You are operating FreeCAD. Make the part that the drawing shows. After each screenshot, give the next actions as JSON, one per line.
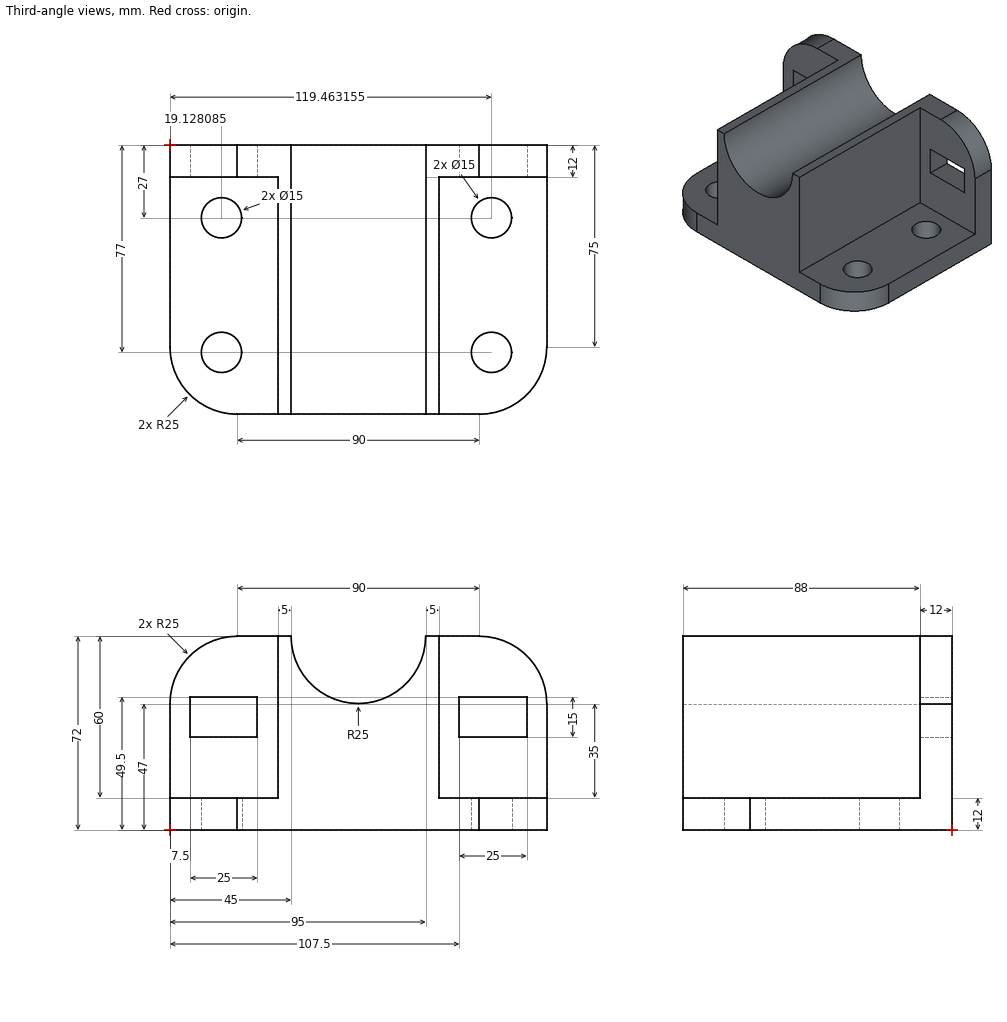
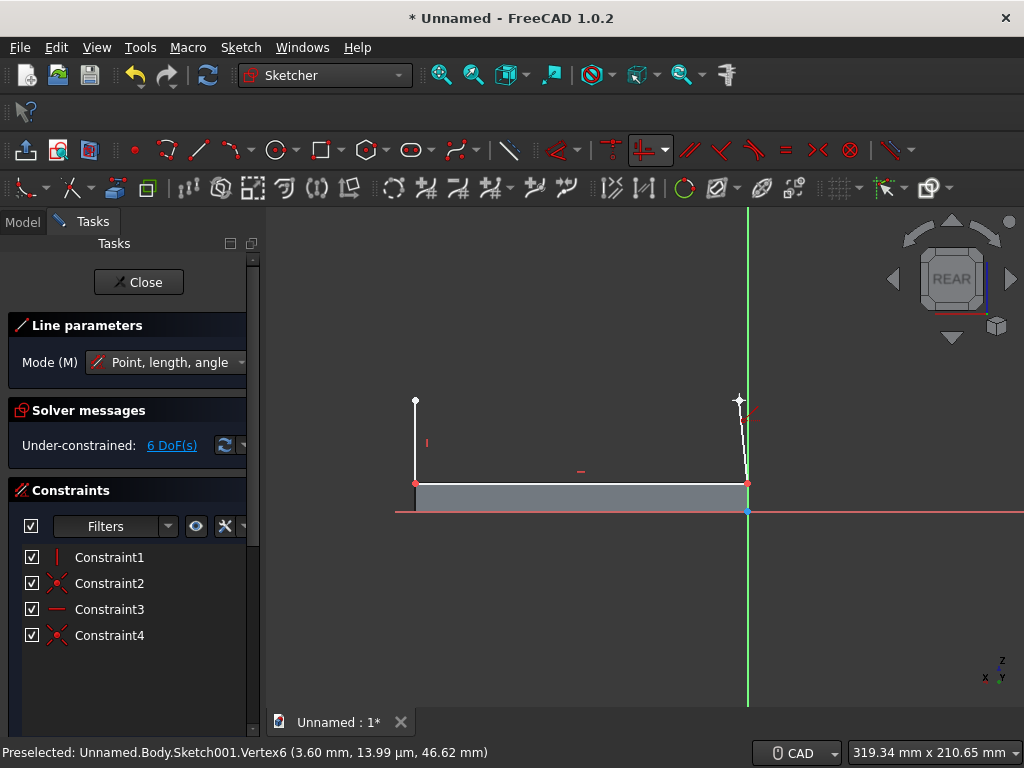
{"action": "left_click", "coordinate": [688, 341]}
{"action": "left_click", "coordinate": [475, 341]}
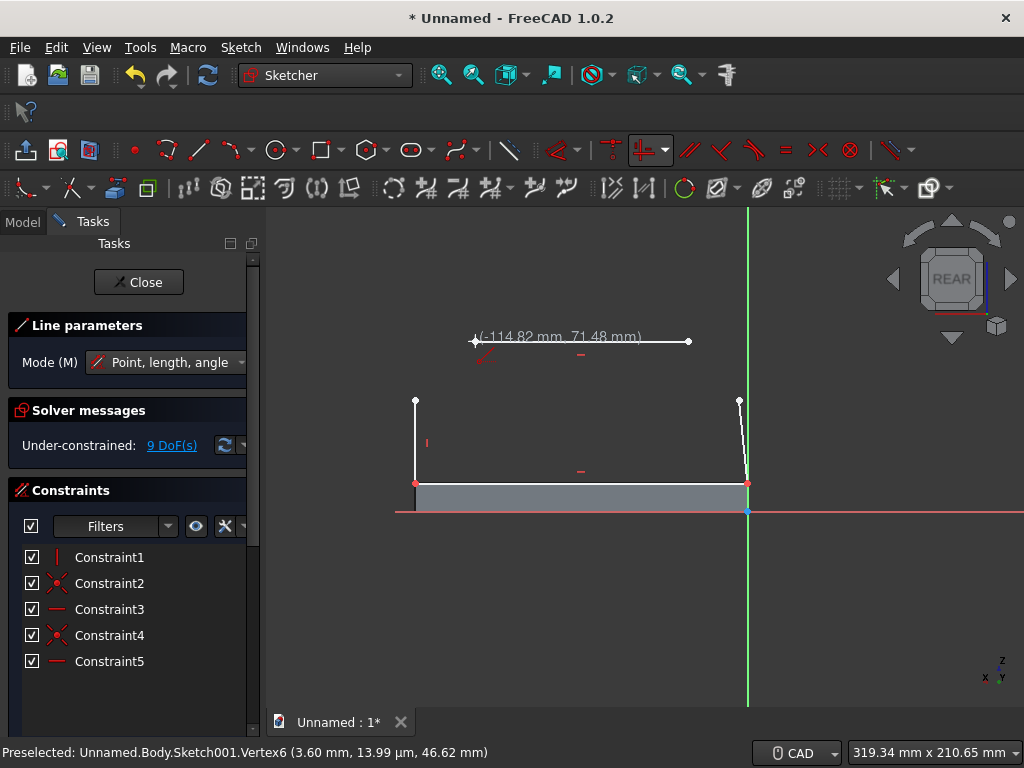
{"action": "left_click", "coordinate": [232, 150]}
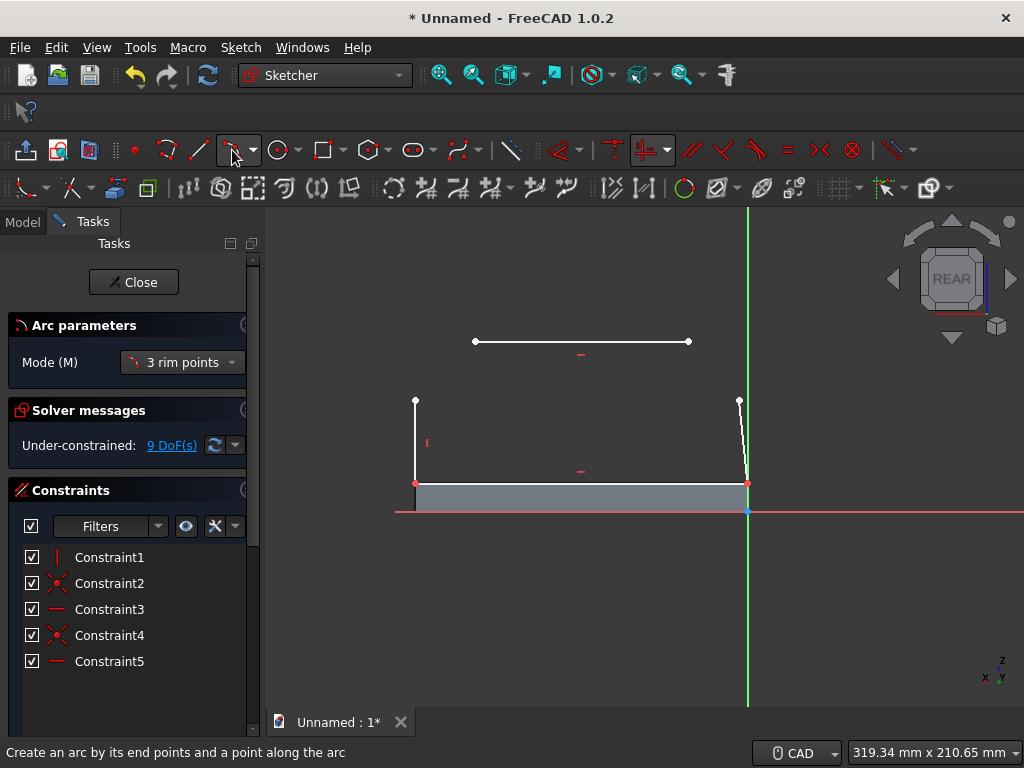
{"action": "left_click", "coordinate": [739, 401]}
{"action": "left_click", "coordinate": [688, 342]}
{"action": "left_click", "coordinate": [730, 358]}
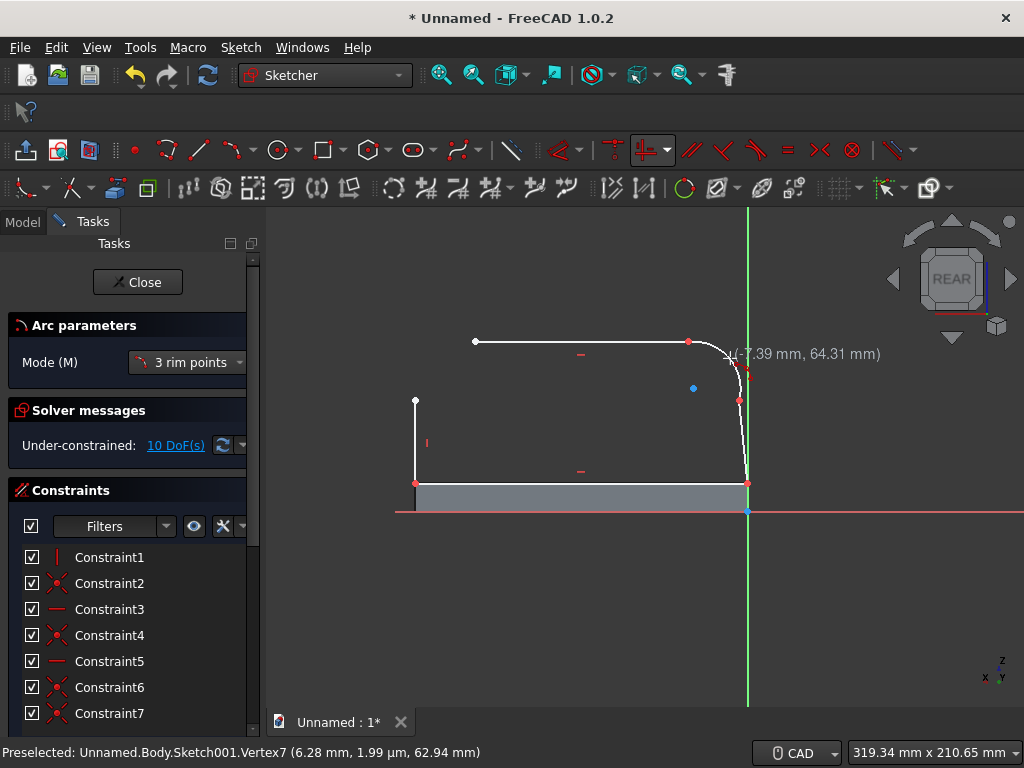
{"action": "left_click", "coordinate": [475, 342]}
{"action": "left_click", "coordinate": [415, 401]}
{"action": "left_click", "coordinate": [433, 358]}
{"action": "key", "text": "Escape"}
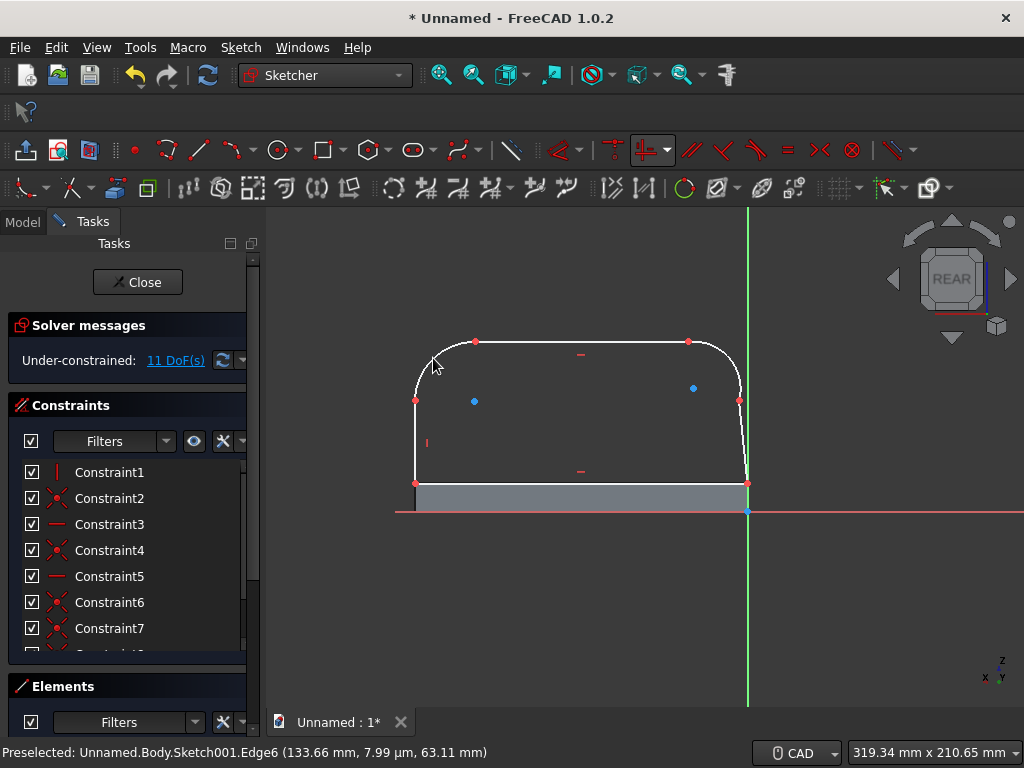
{"action": "left_click", "coordinate": [415, 426]}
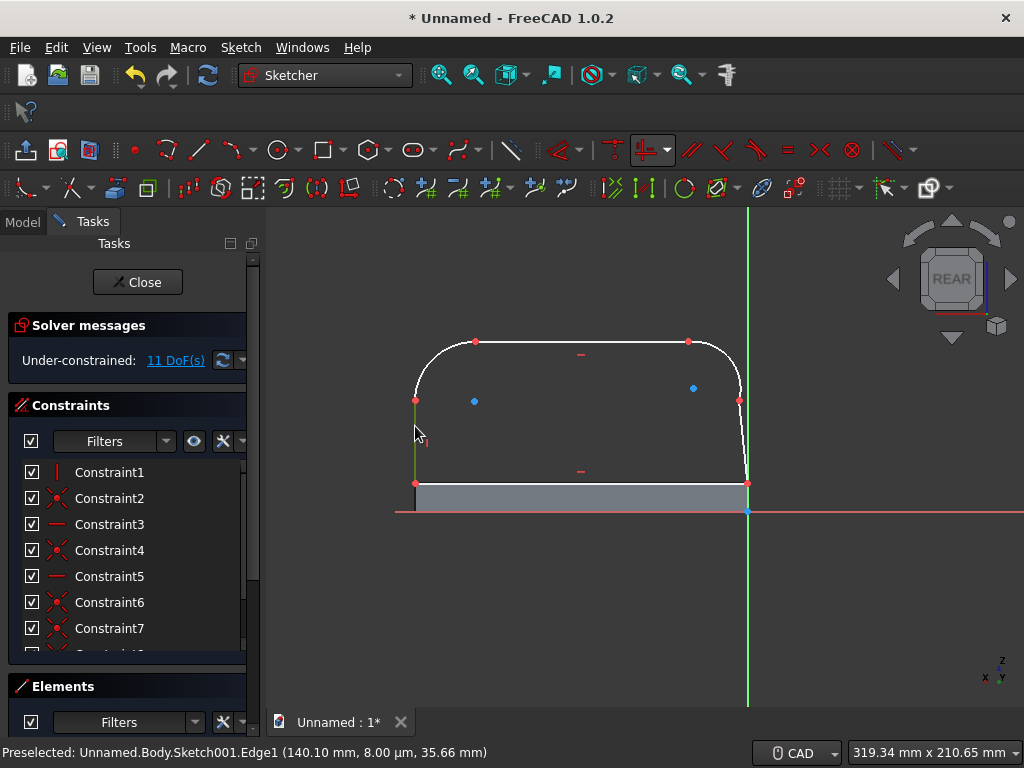
{"action": "left_click", "coordinate": [448, 348]}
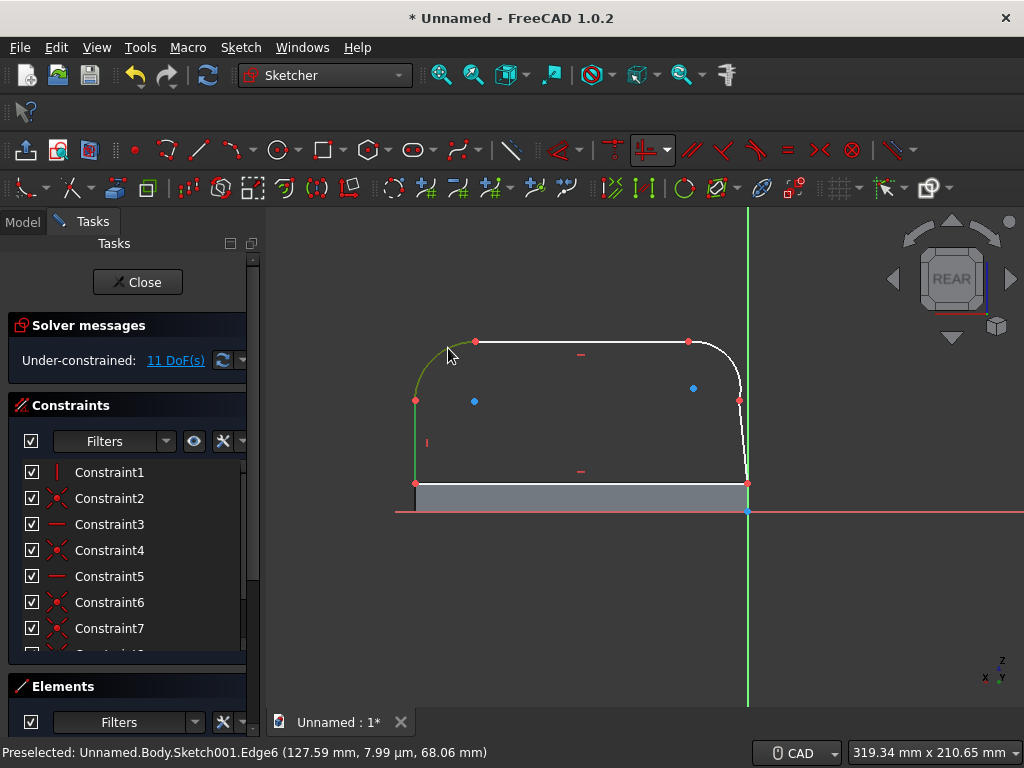
{"action": "key", "text": "t"}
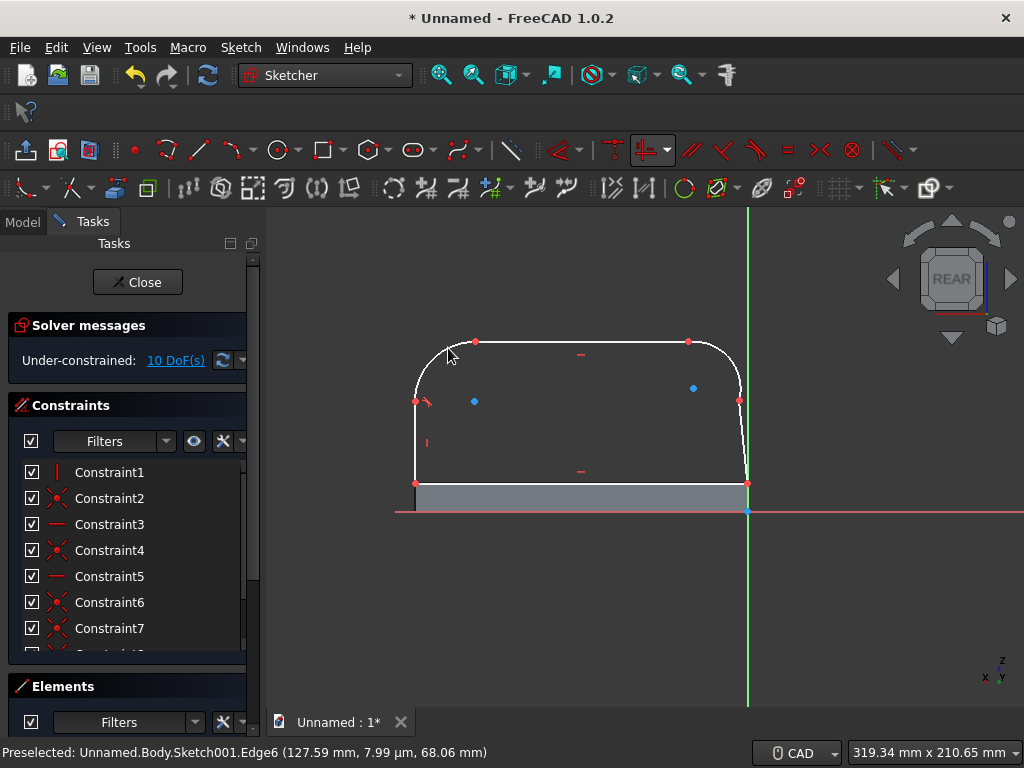
{"action": "left_click", "coordinate": [745, 459]}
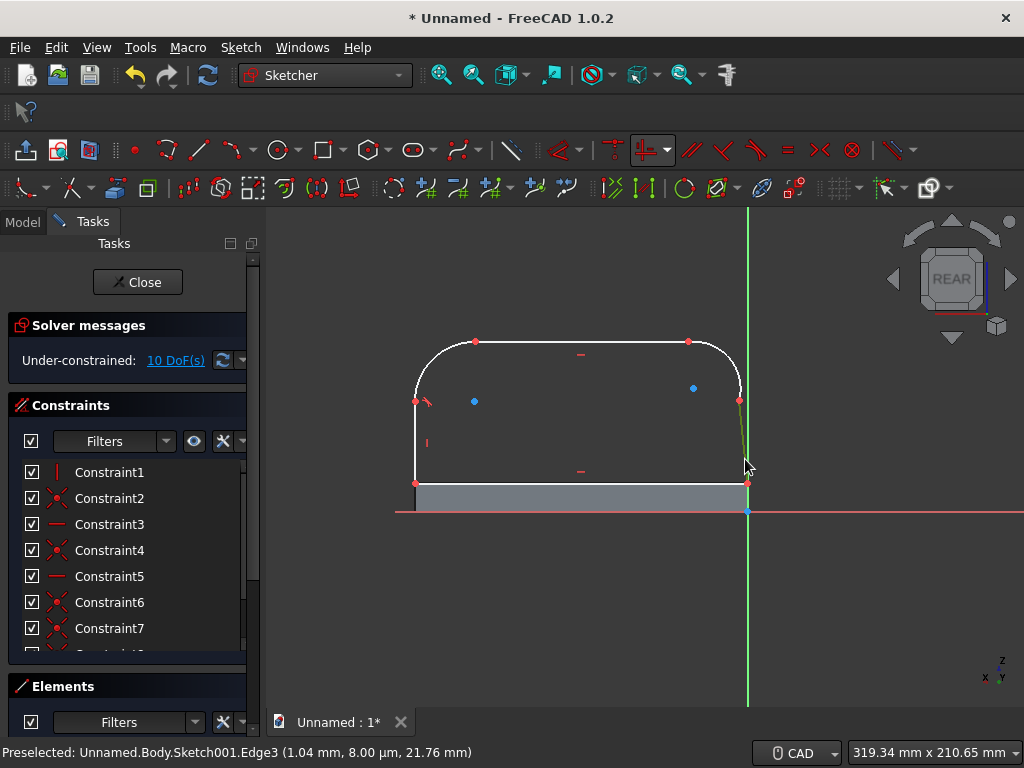
{"action": "scroll", "coordinate": [738, 374], "scroll_direction": "up", "scroll_amount": 2}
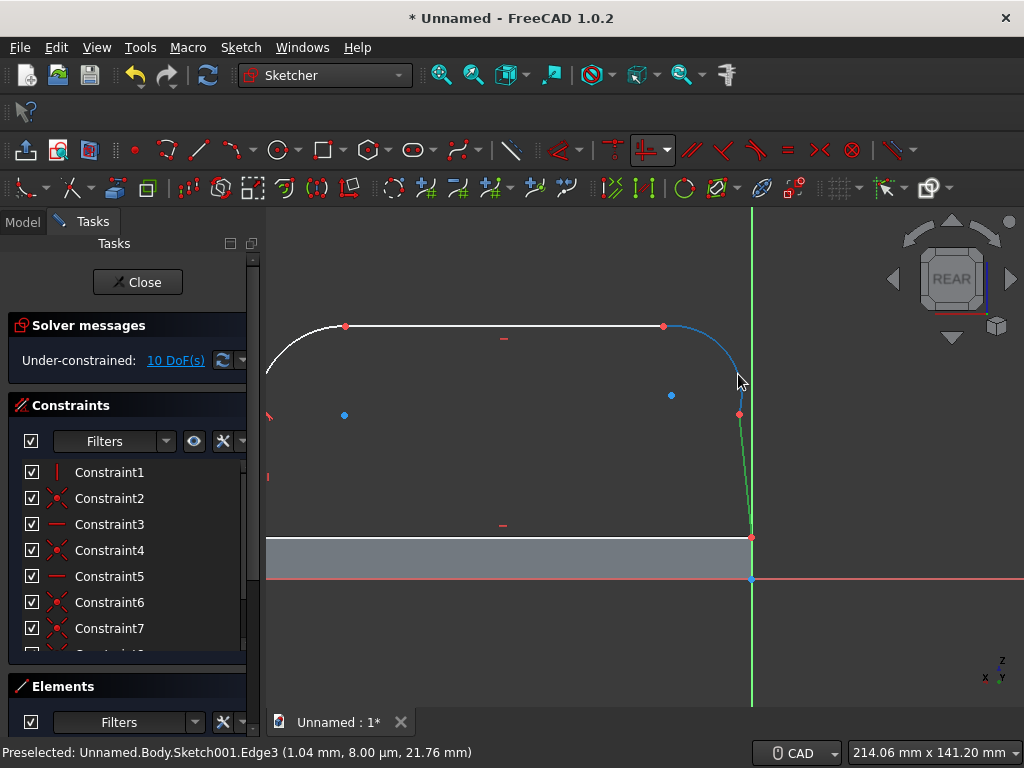
{"action": "left_click", "coordinate": [738, 374]}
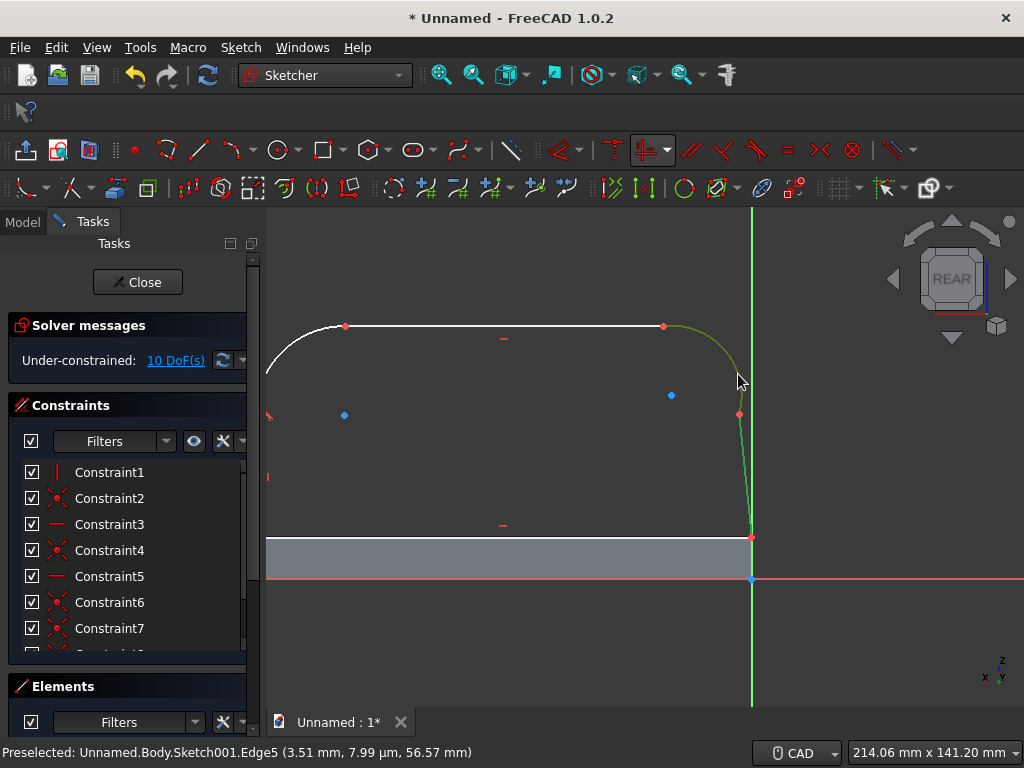
{"action": "left_click", "coordinate": [756, 150]}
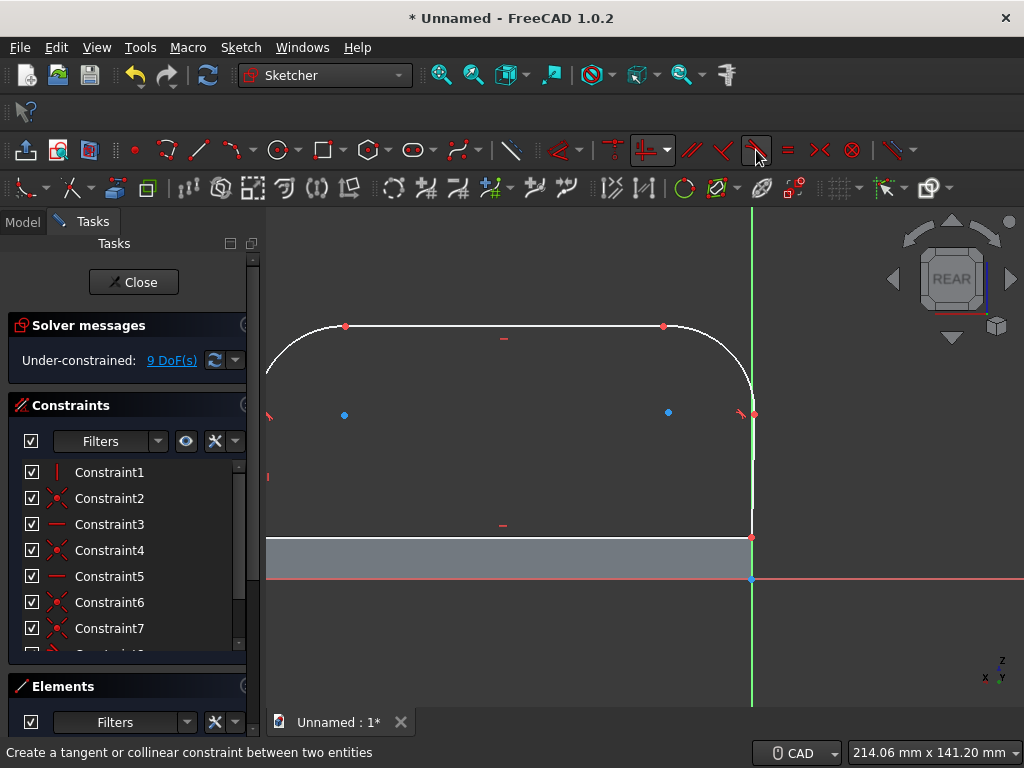
{"action": "left_click", "coordinate": [568, 326]}